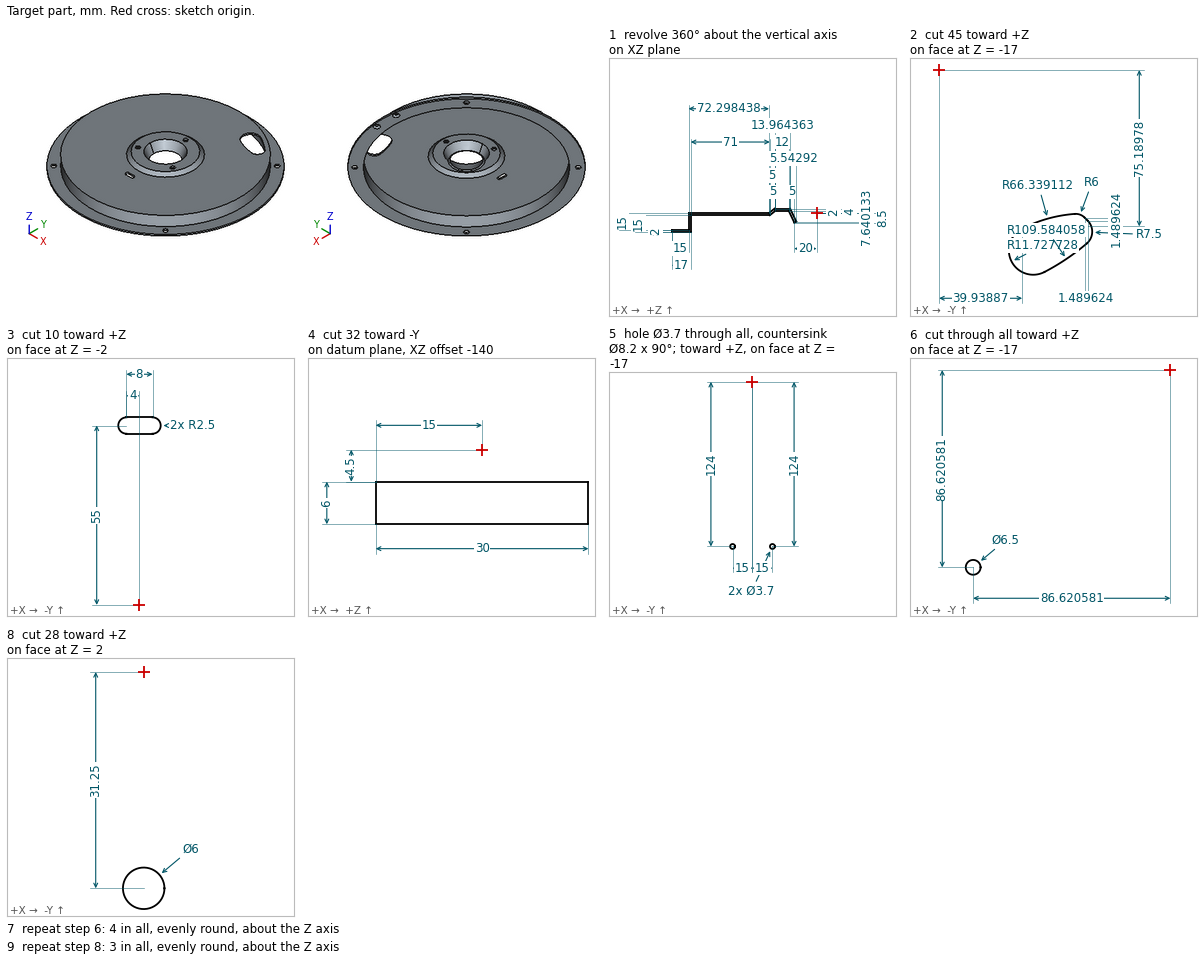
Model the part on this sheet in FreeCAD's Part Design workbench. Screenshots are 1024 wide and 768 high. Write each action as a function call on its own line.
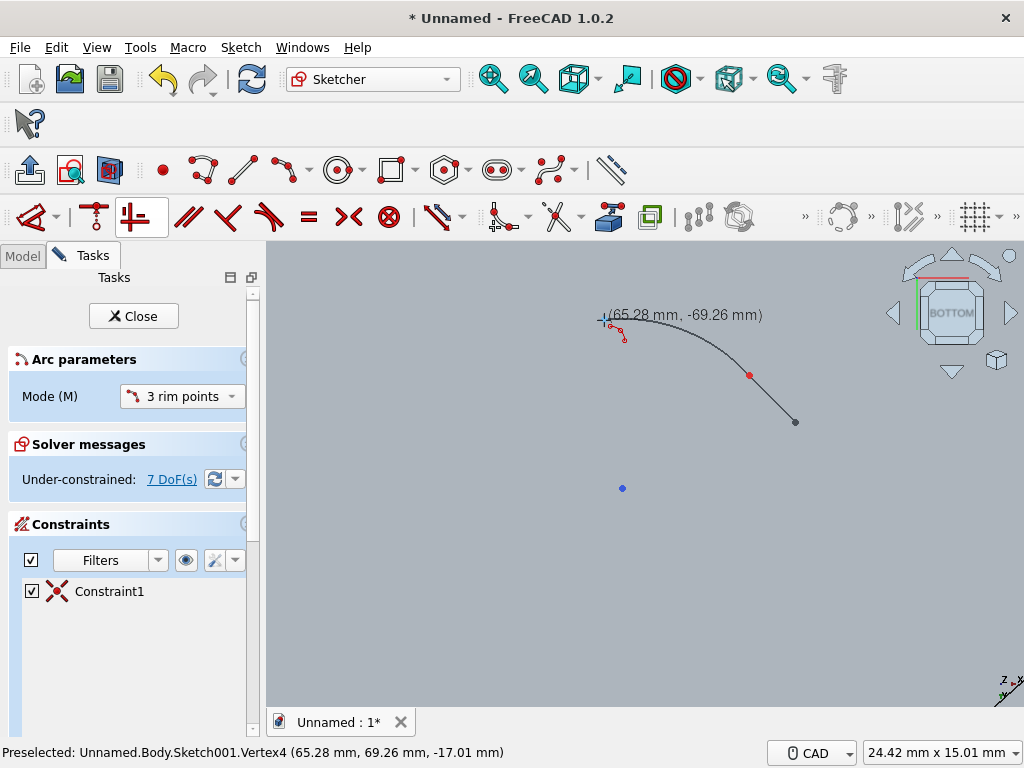
scroll(712, 354, down, 6)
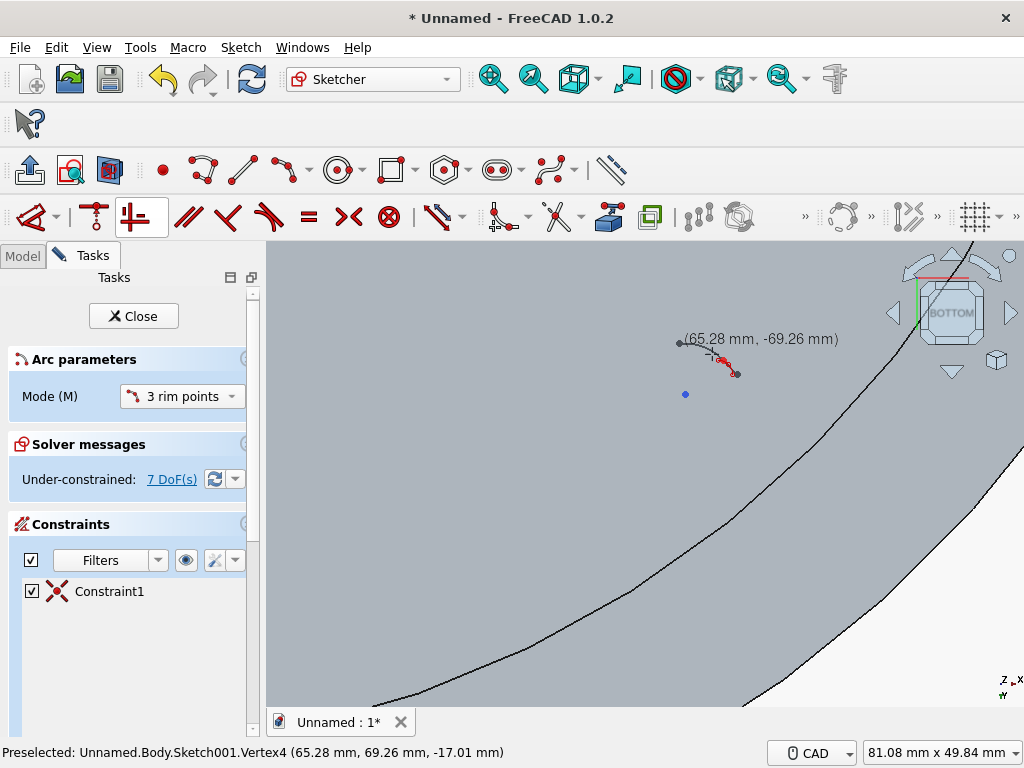
click(443, 410)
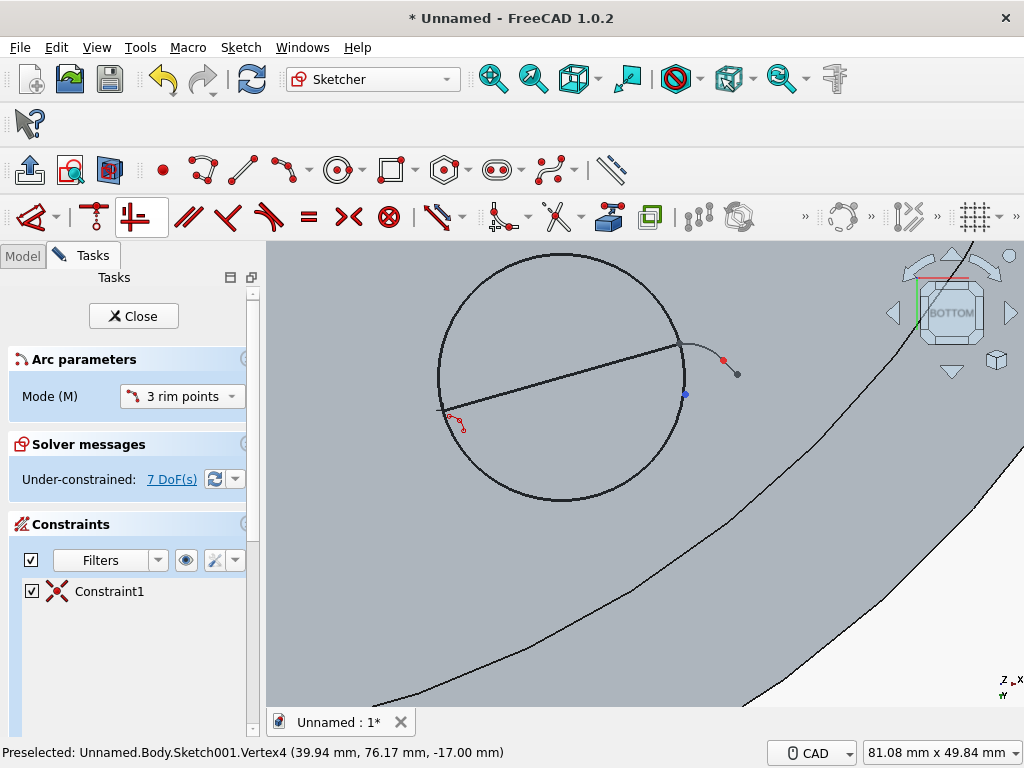
scroll(558, 365, up, 2)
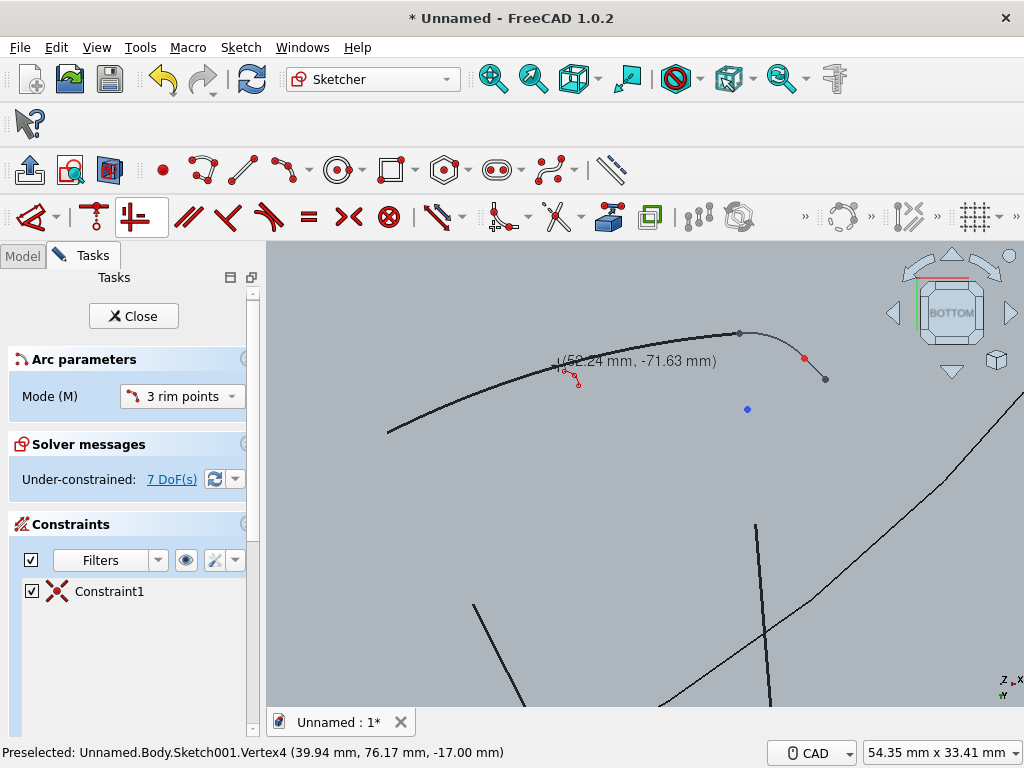
click(558, 364)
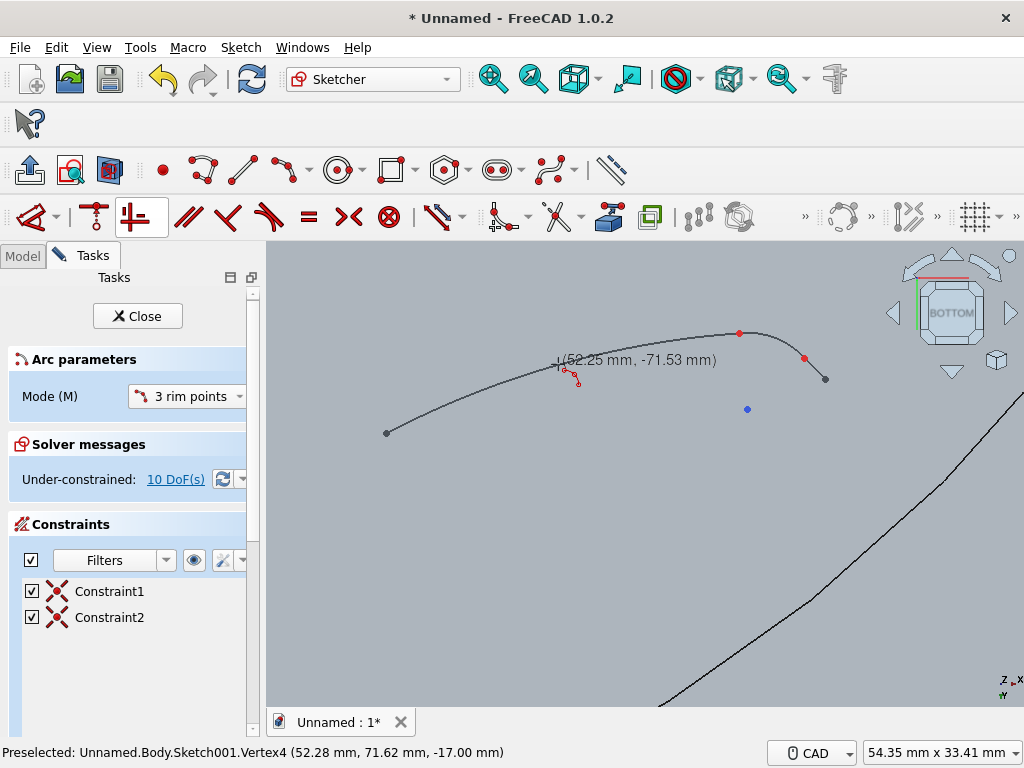
click(386, 433)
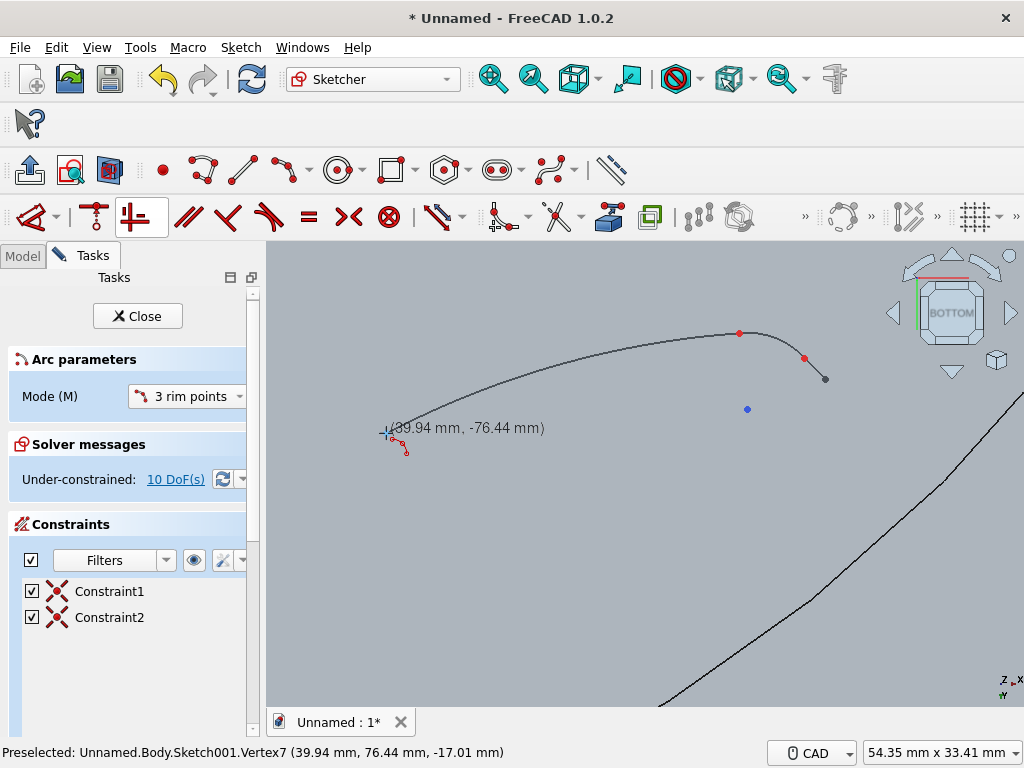
scroll(557, 365, down, 2)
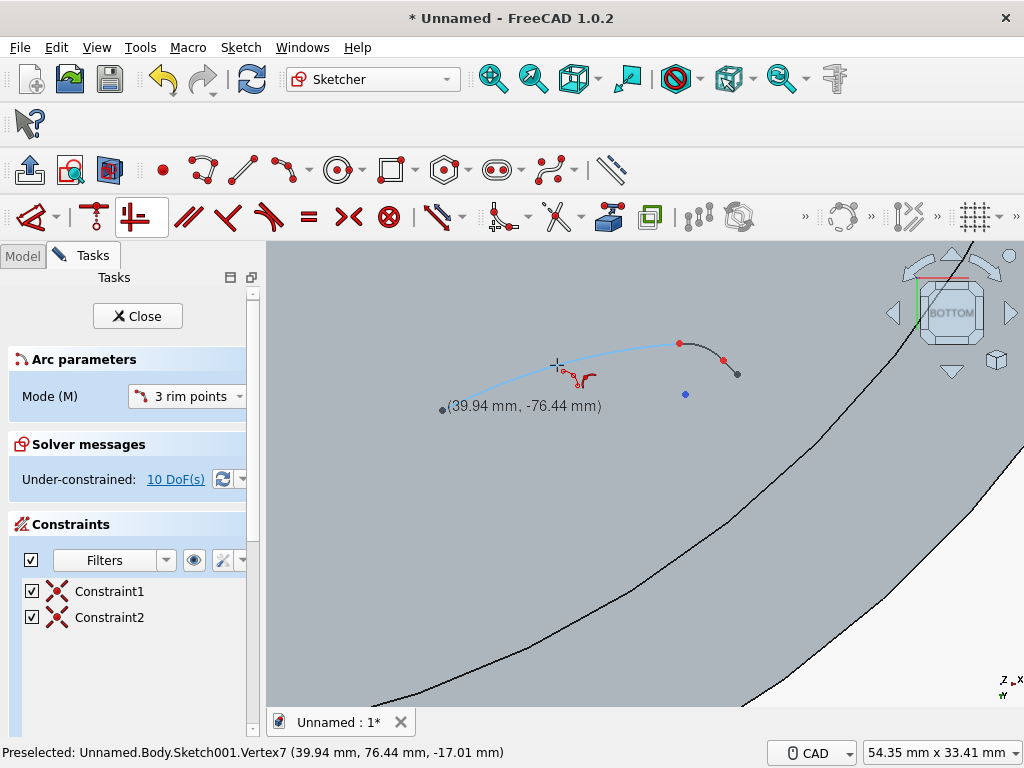
click(543, 605)
click(395, 558)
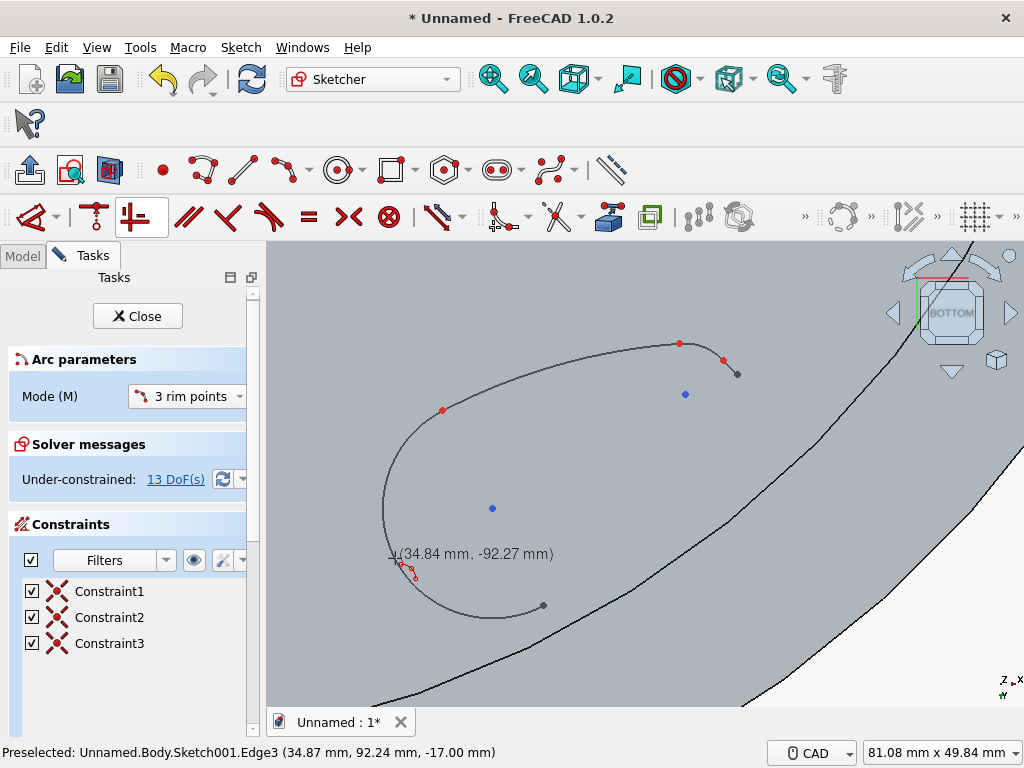
click(543, 606)
click(733, 477)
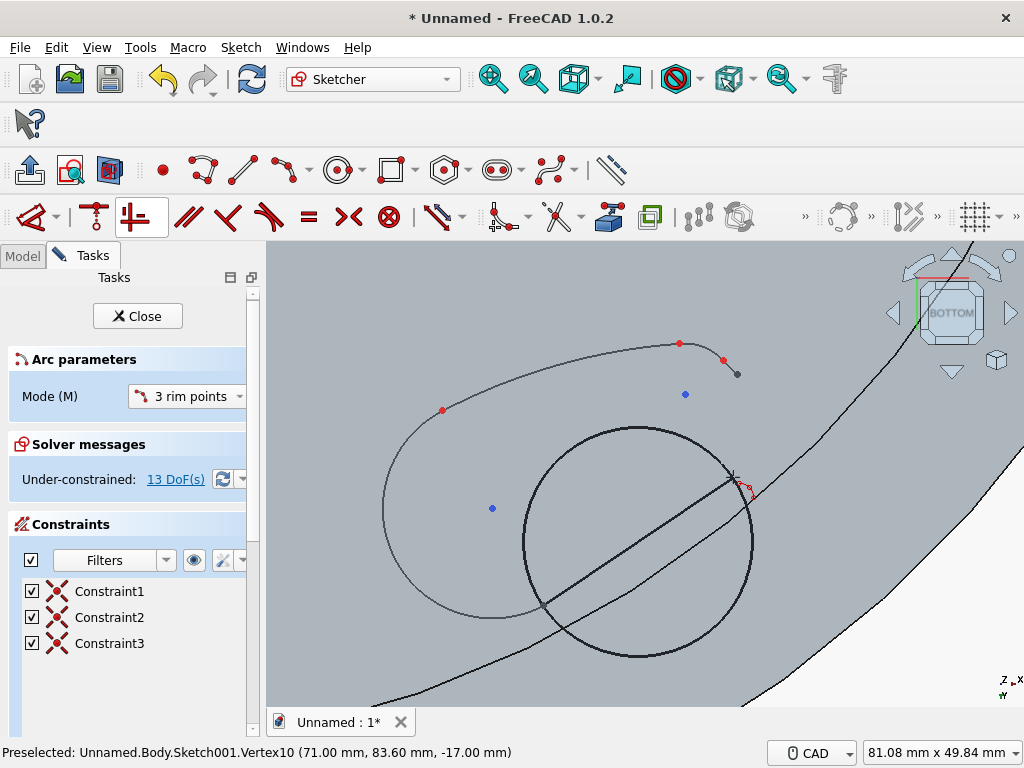
scroll(642, 546, up, 5)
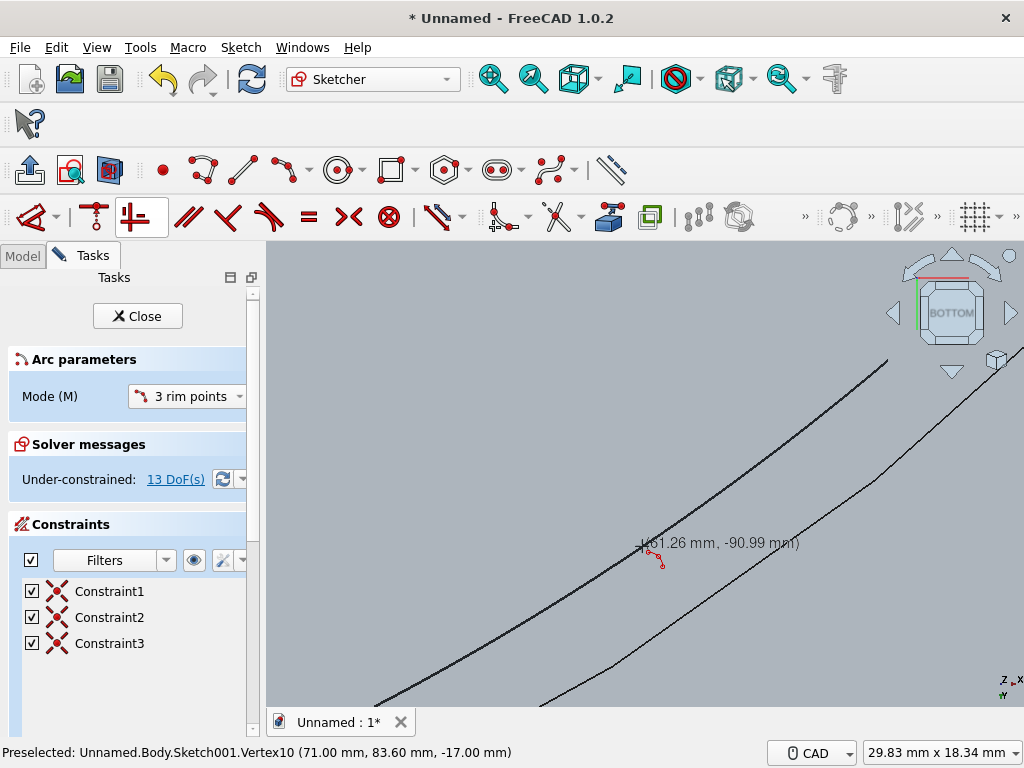
click(641, 545)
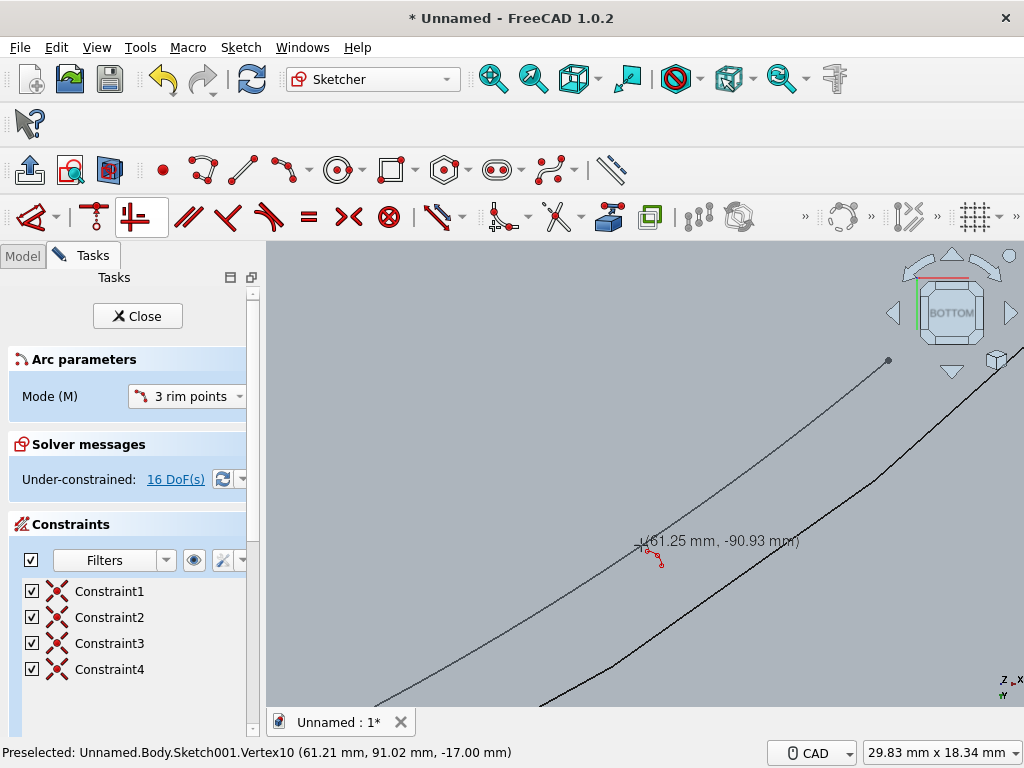
scroll(642, 547, down, 5)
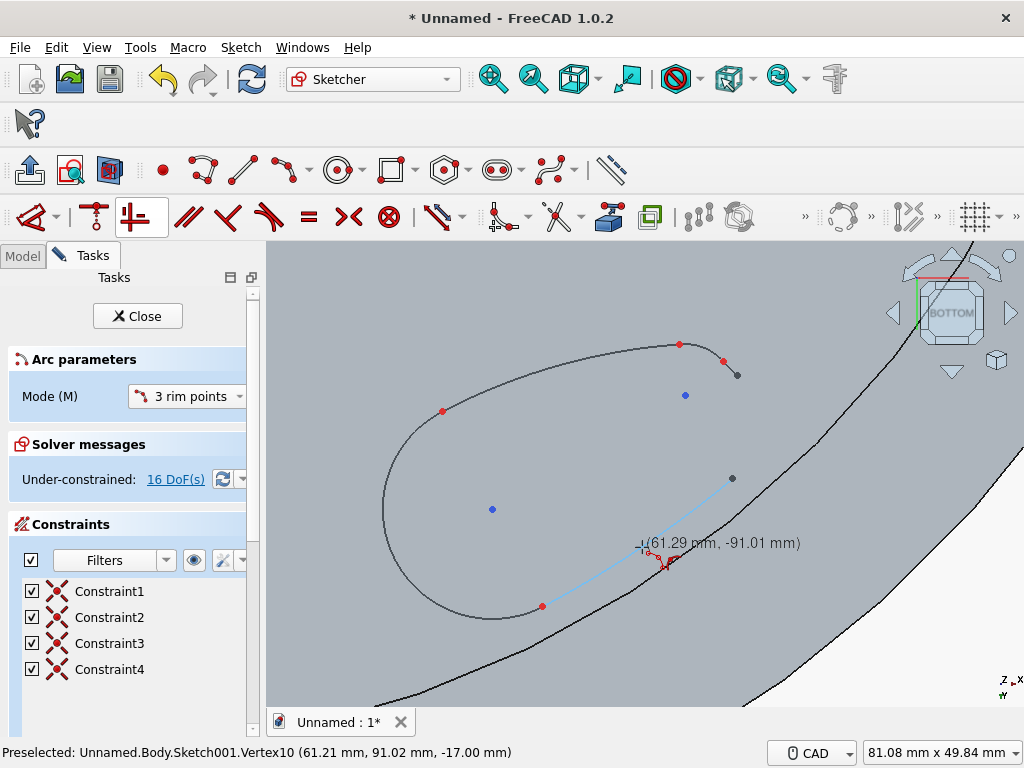
click(733, 479)